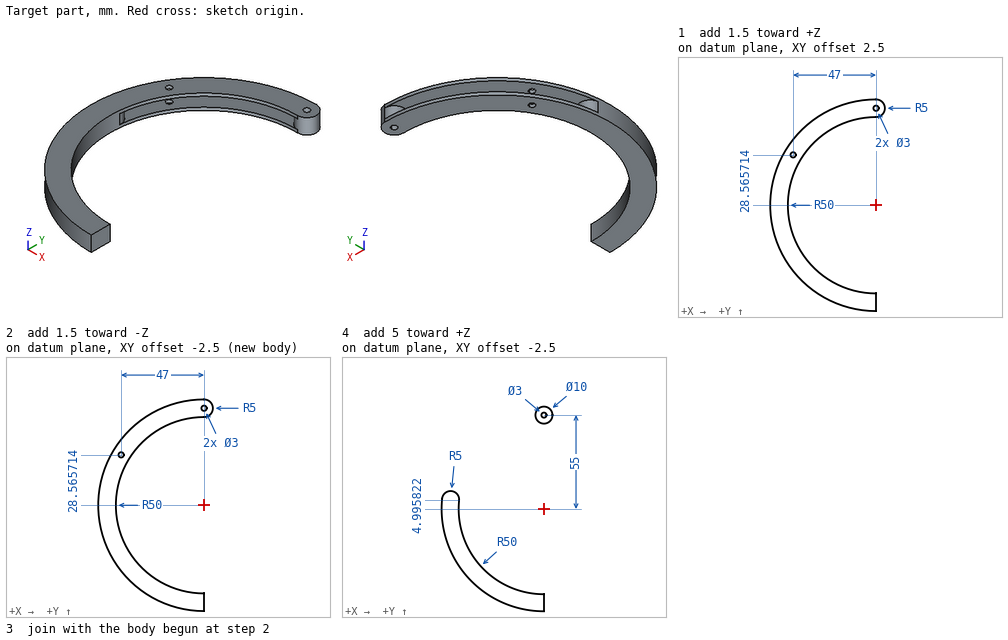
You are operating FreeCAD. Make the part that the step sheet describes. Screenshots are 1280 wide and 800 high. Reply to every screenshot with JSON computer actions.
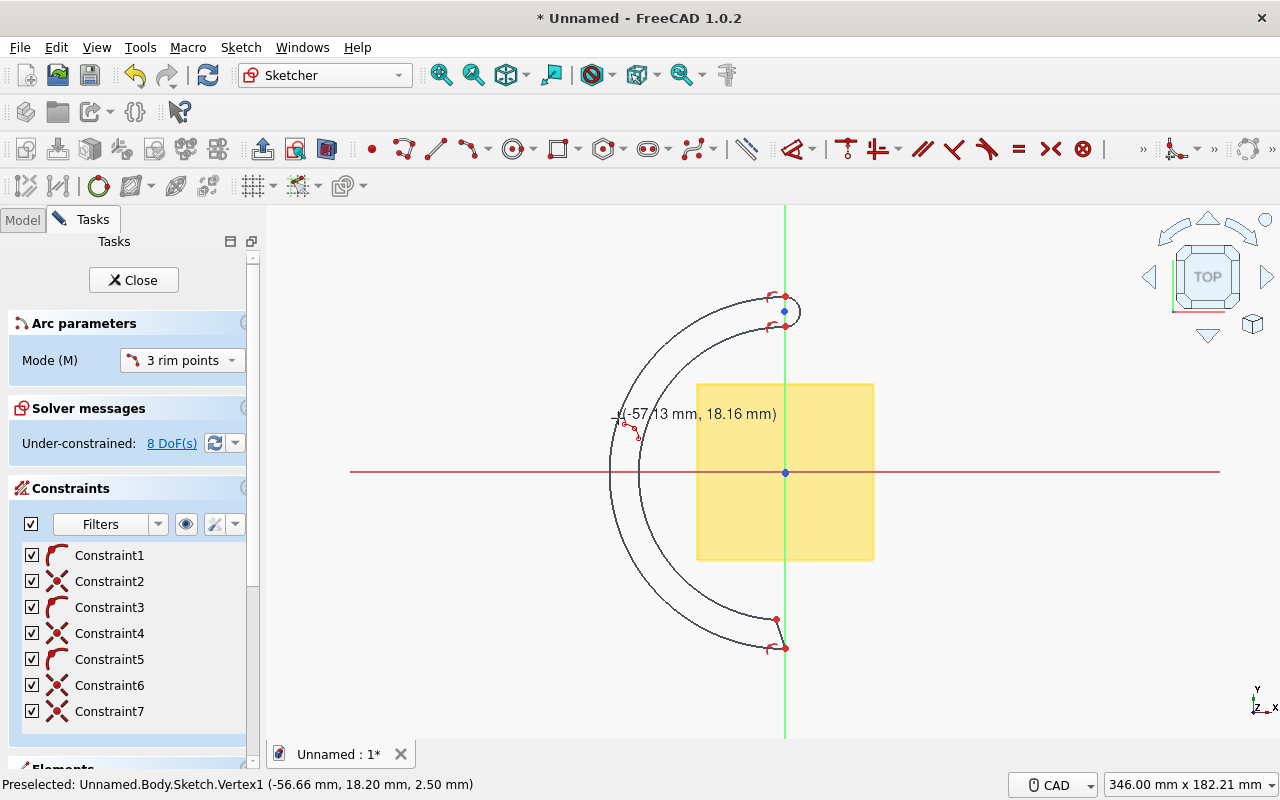
{"action": "left_click", "coordinate": [514, 150]}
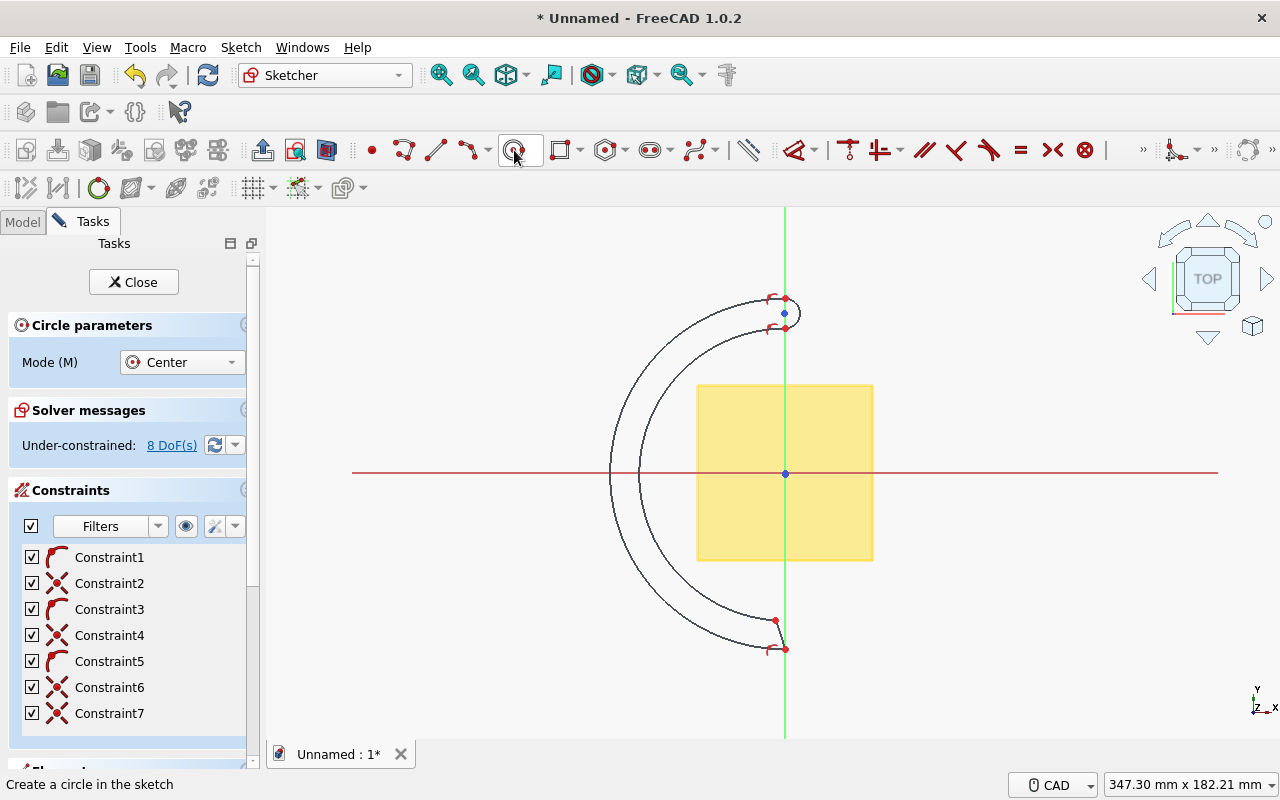
{"action": "scroll", "coordinate": [648, 390], "scroll_direction": "up", "scroll_amount": 9}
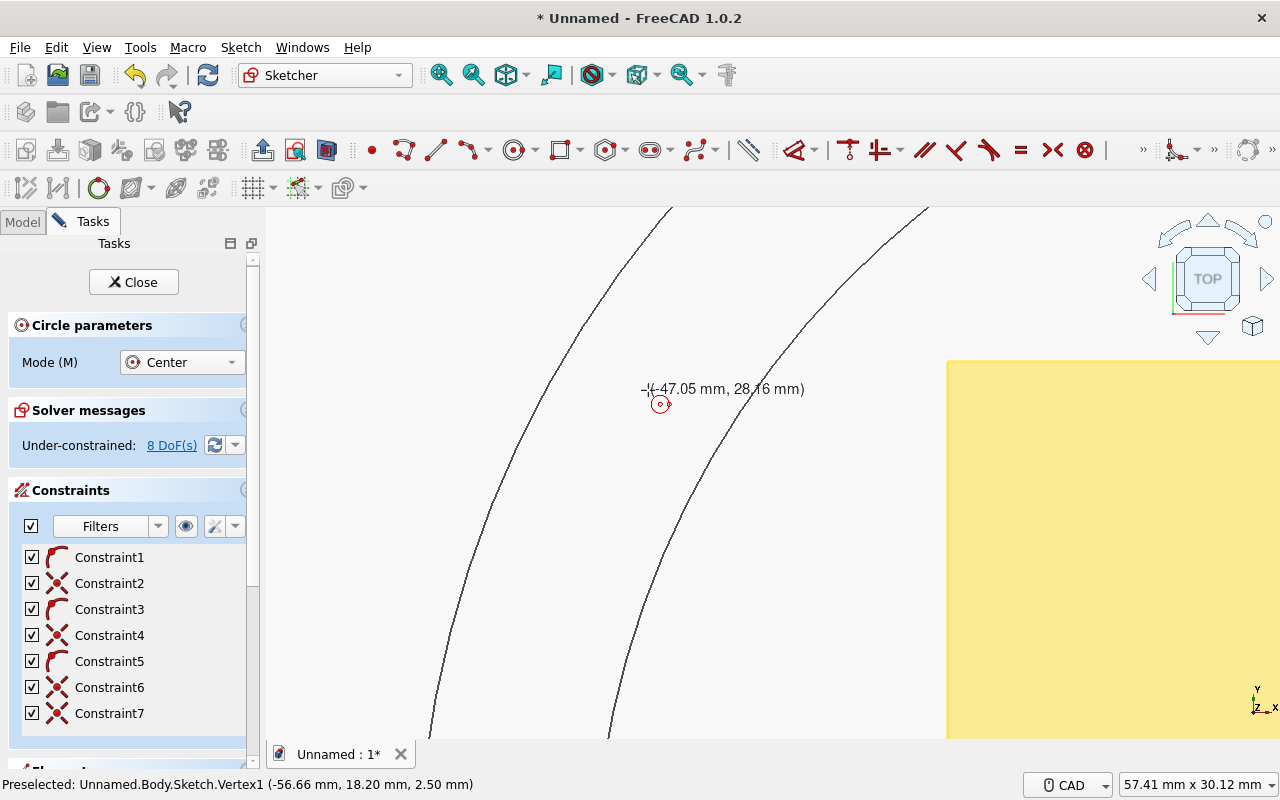
{"action": "scroll", "coordinate": [648, 390], "scroll_direction": "down", "scroll_amount": 9}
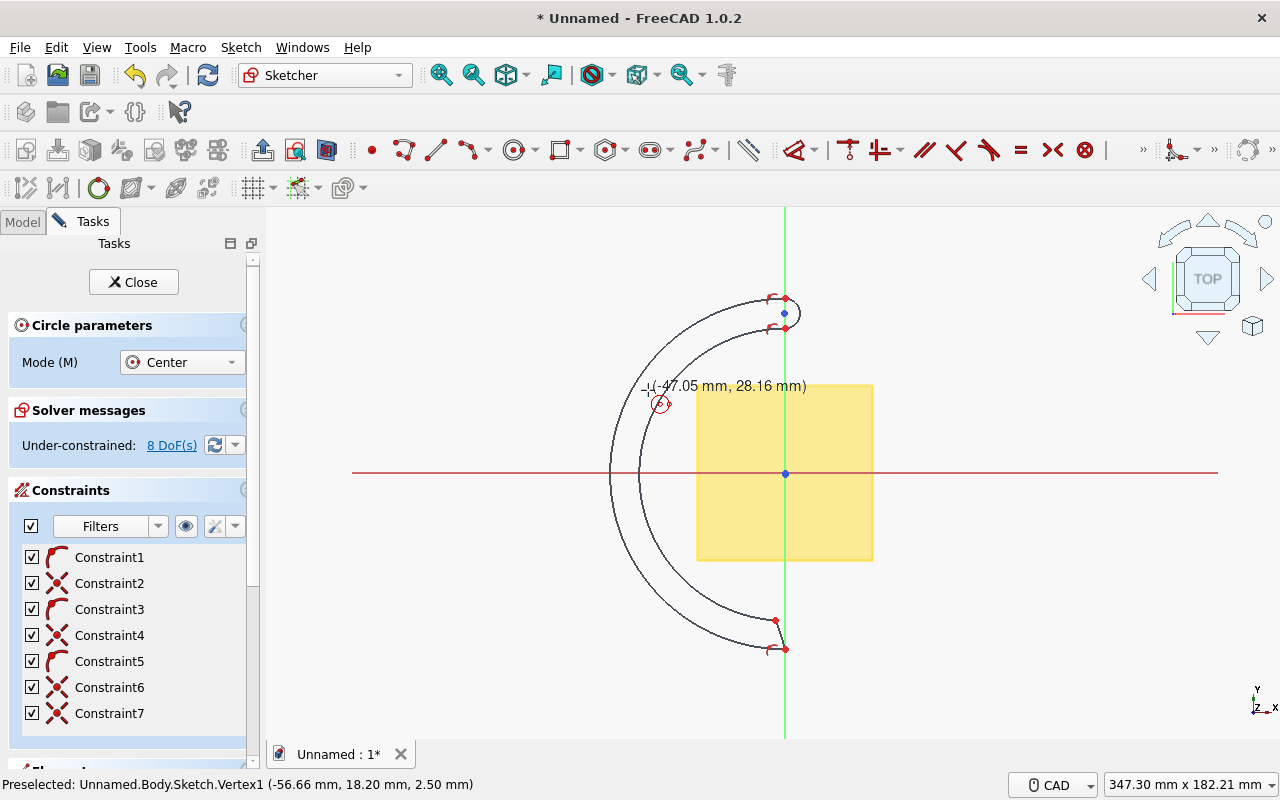
{"action": "left_click", "coordinate": [648, 390]}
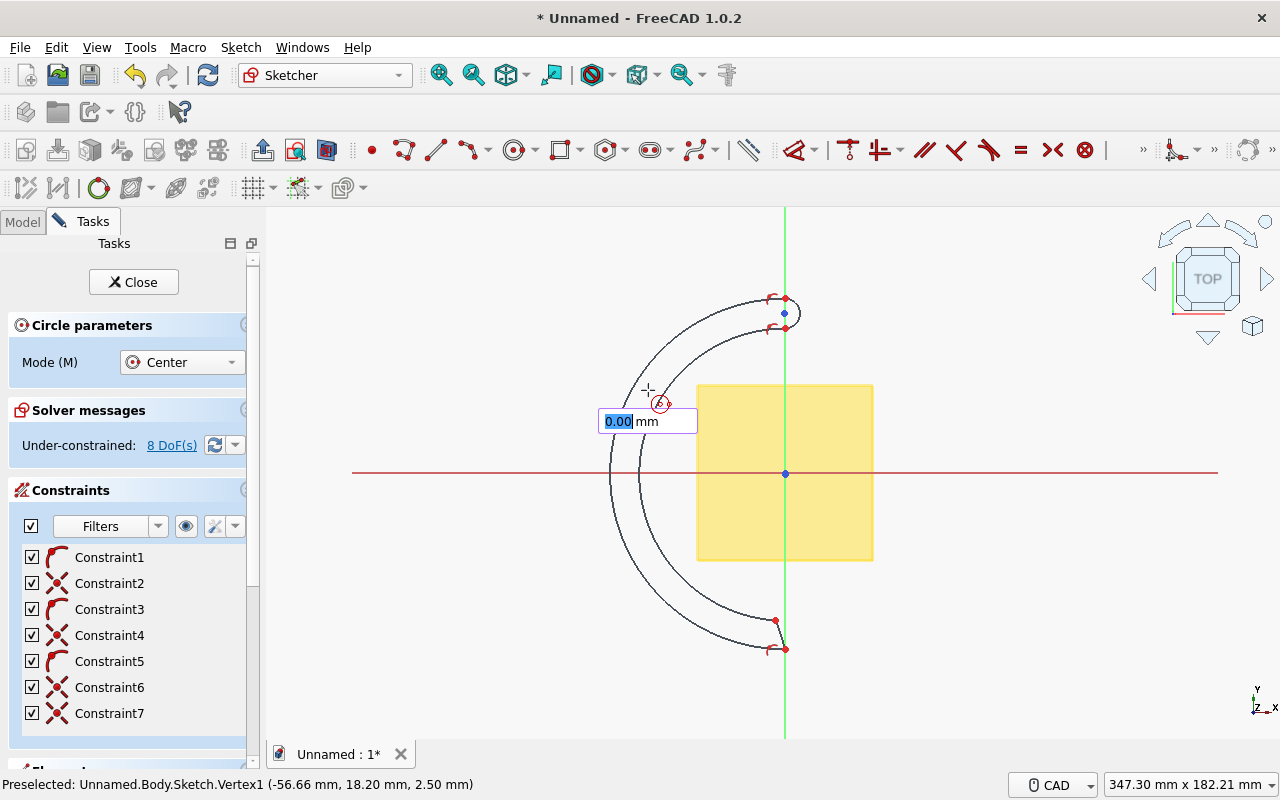
{"action": "scroll", "coordinate": [647, 394], "scroll_direction": "up", "scroll_amount": 7}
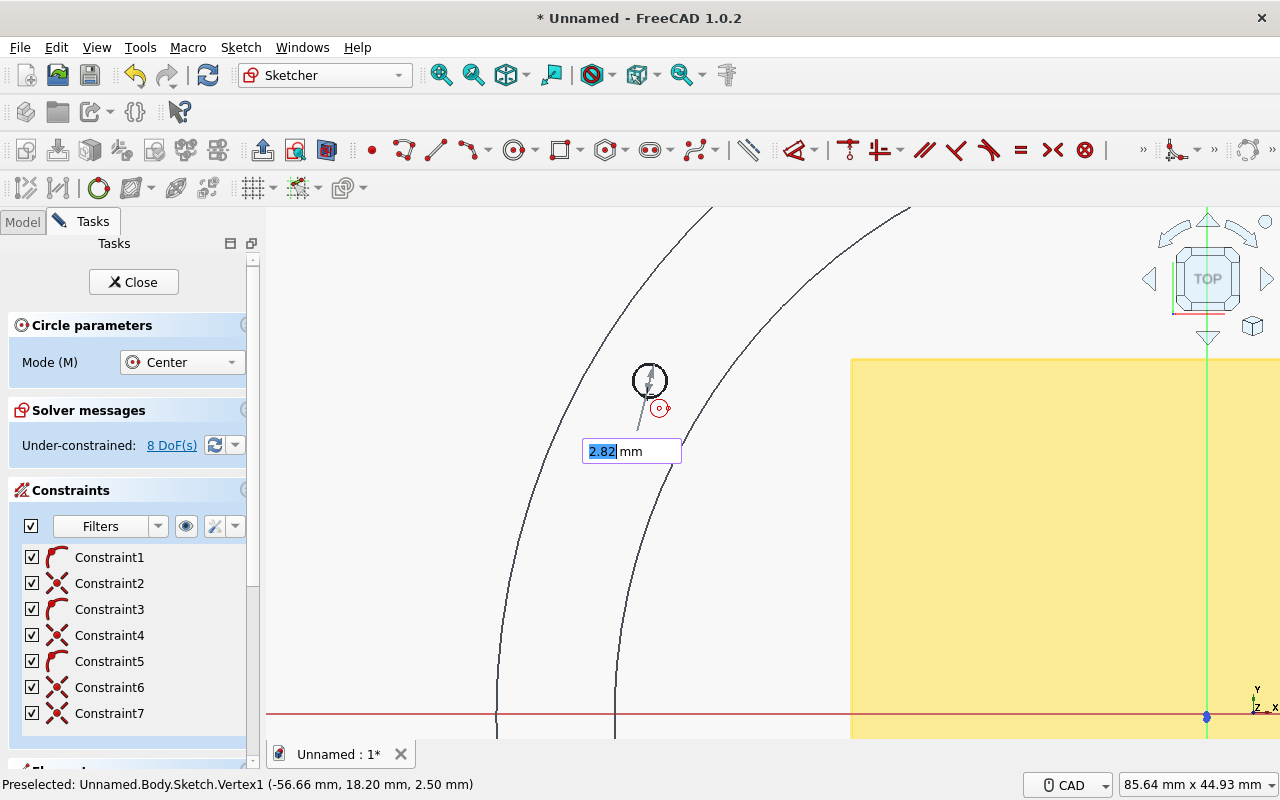
{"action": "left_click", "coordinate": [644, 393]}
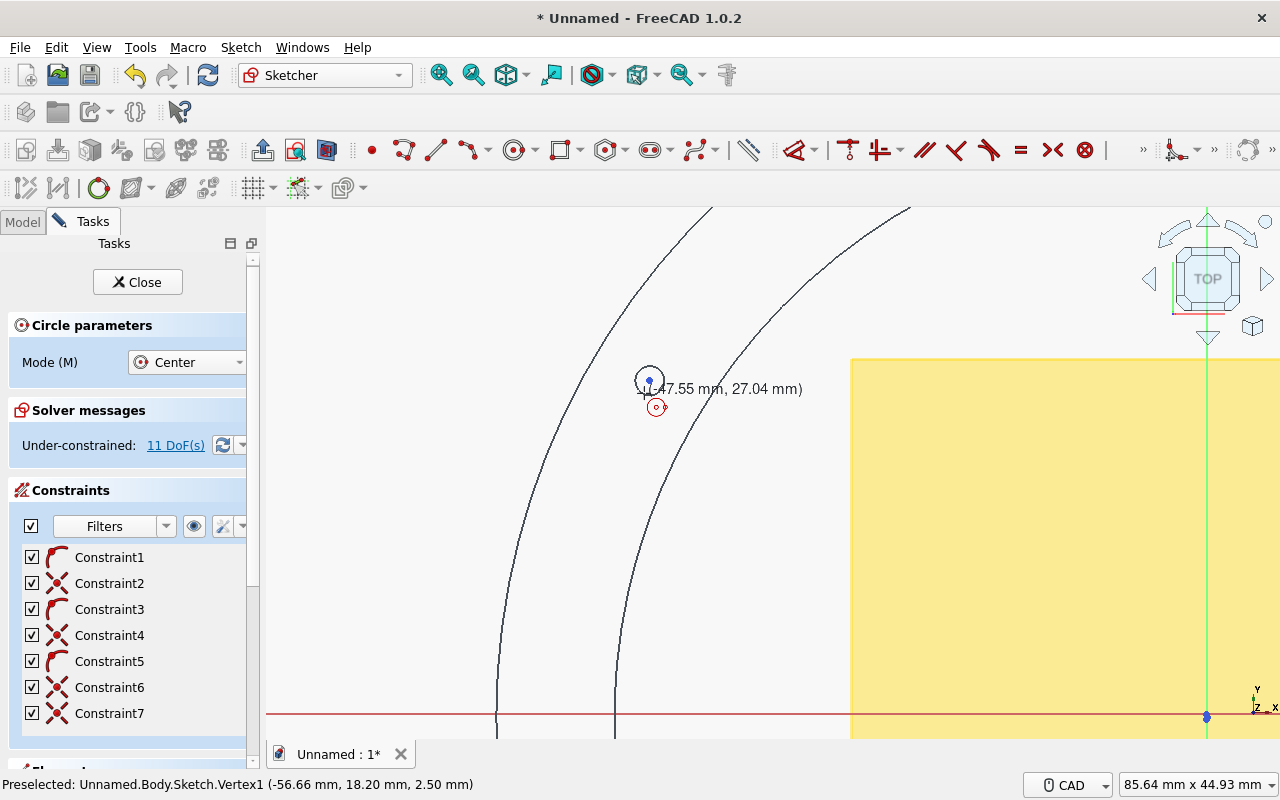
{"action": "scroll", "coordinate": [647, 394], "scroll_direction": "down", "scroll_amount": 7}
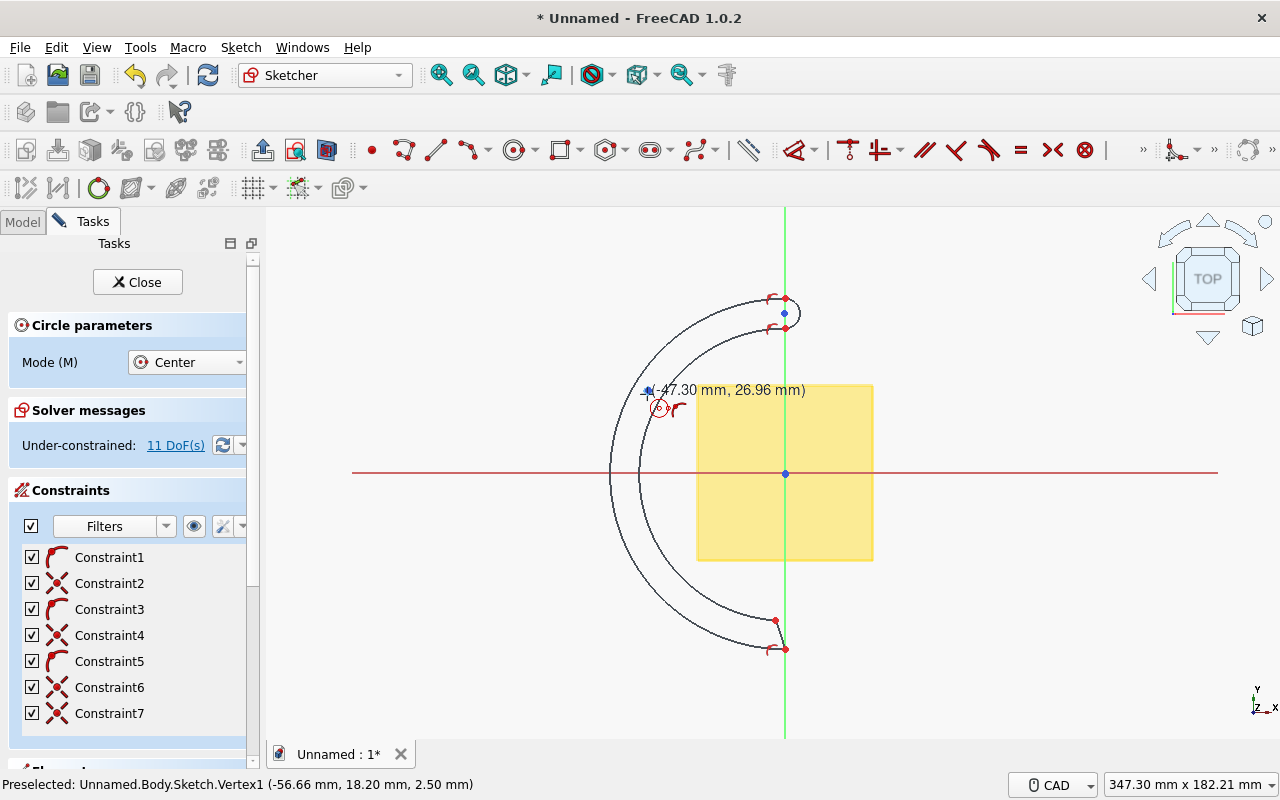
{"action": "scroll", "coordinate": [785, 313], "scroll_direction": "up", "scroll_amount": 9}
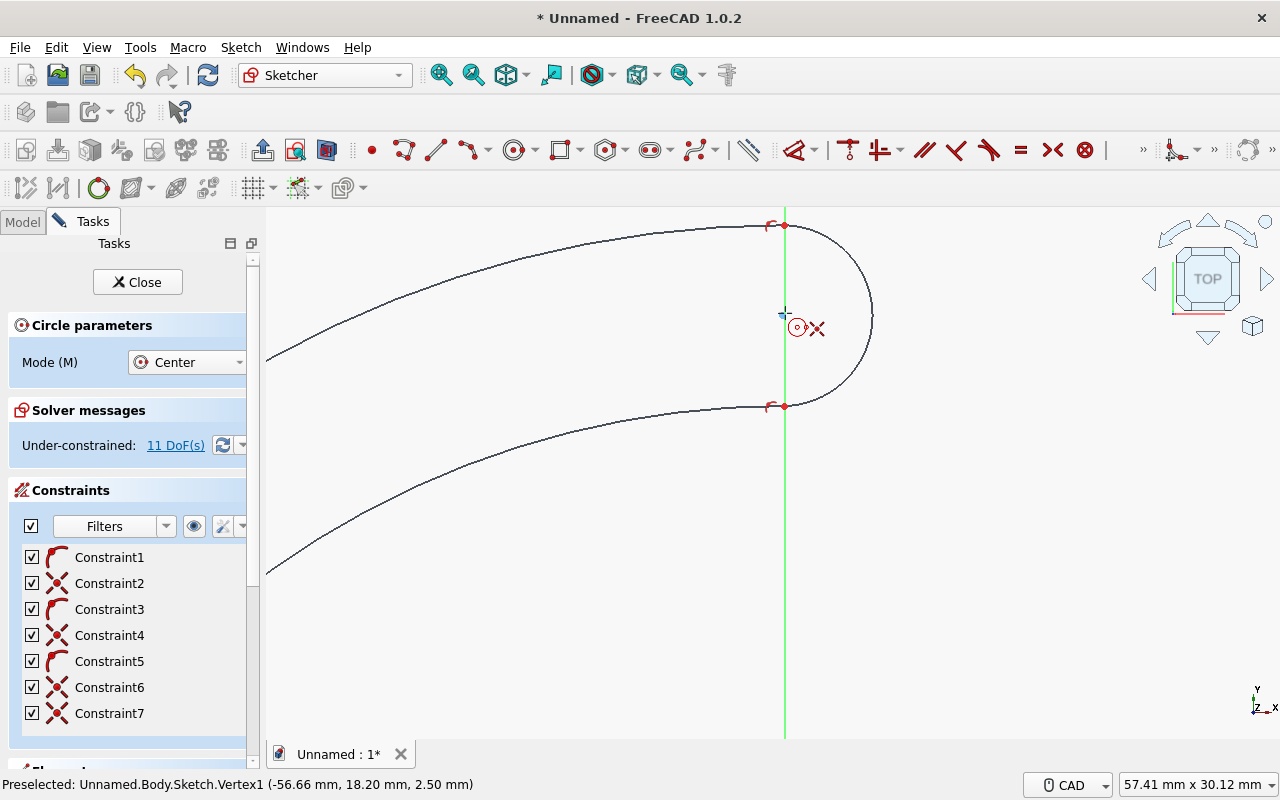
{"action": "scroll", "coordinate": [785, 313], "scroll_direction": "down", "scroll_amount": 9}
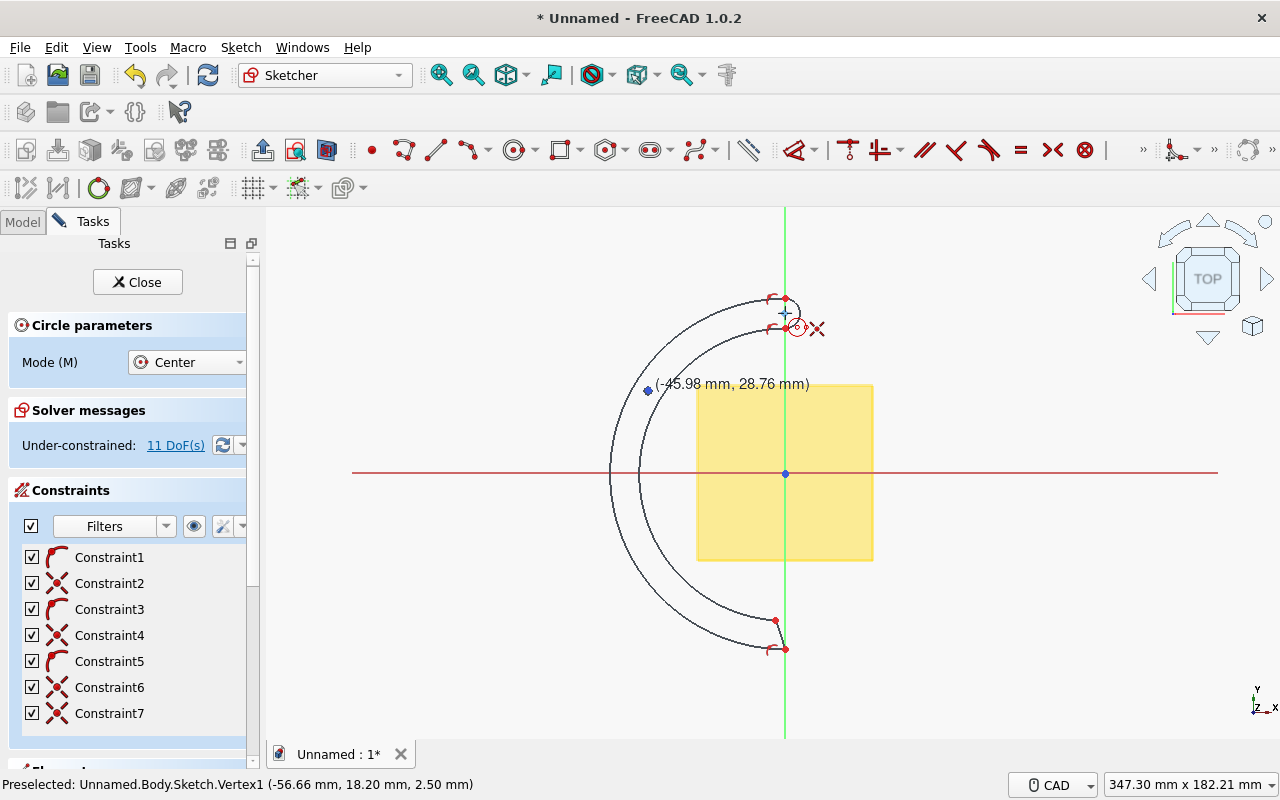
{"action": "left_click", "coordinate": [785, 313]}